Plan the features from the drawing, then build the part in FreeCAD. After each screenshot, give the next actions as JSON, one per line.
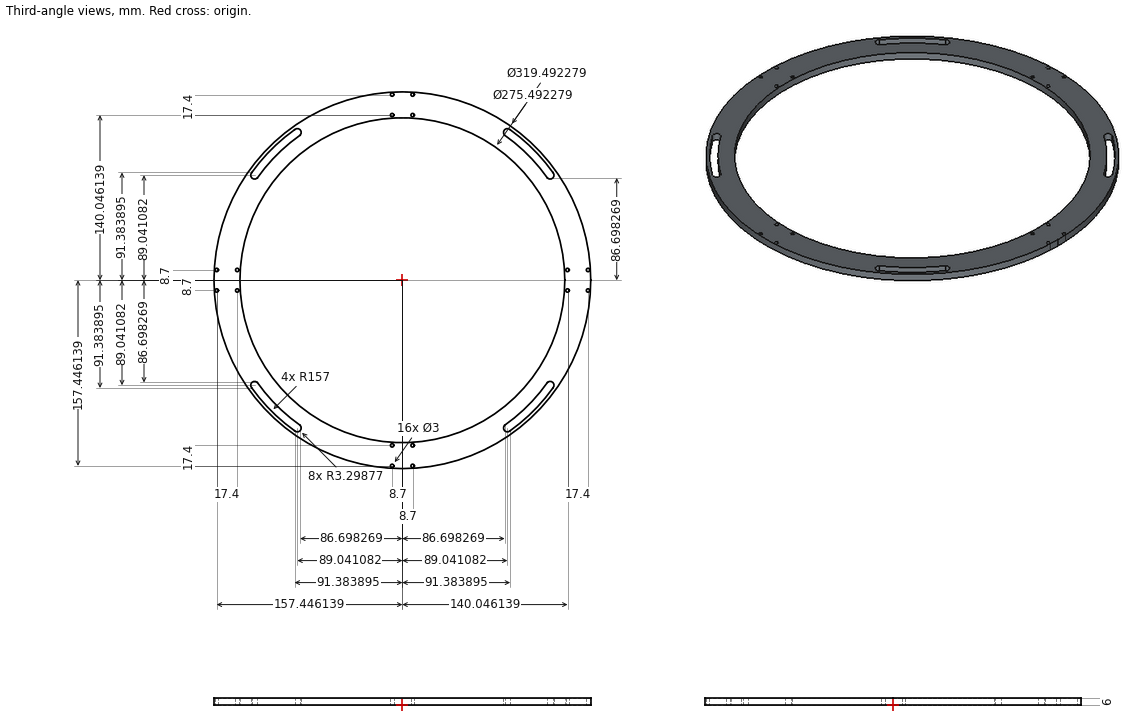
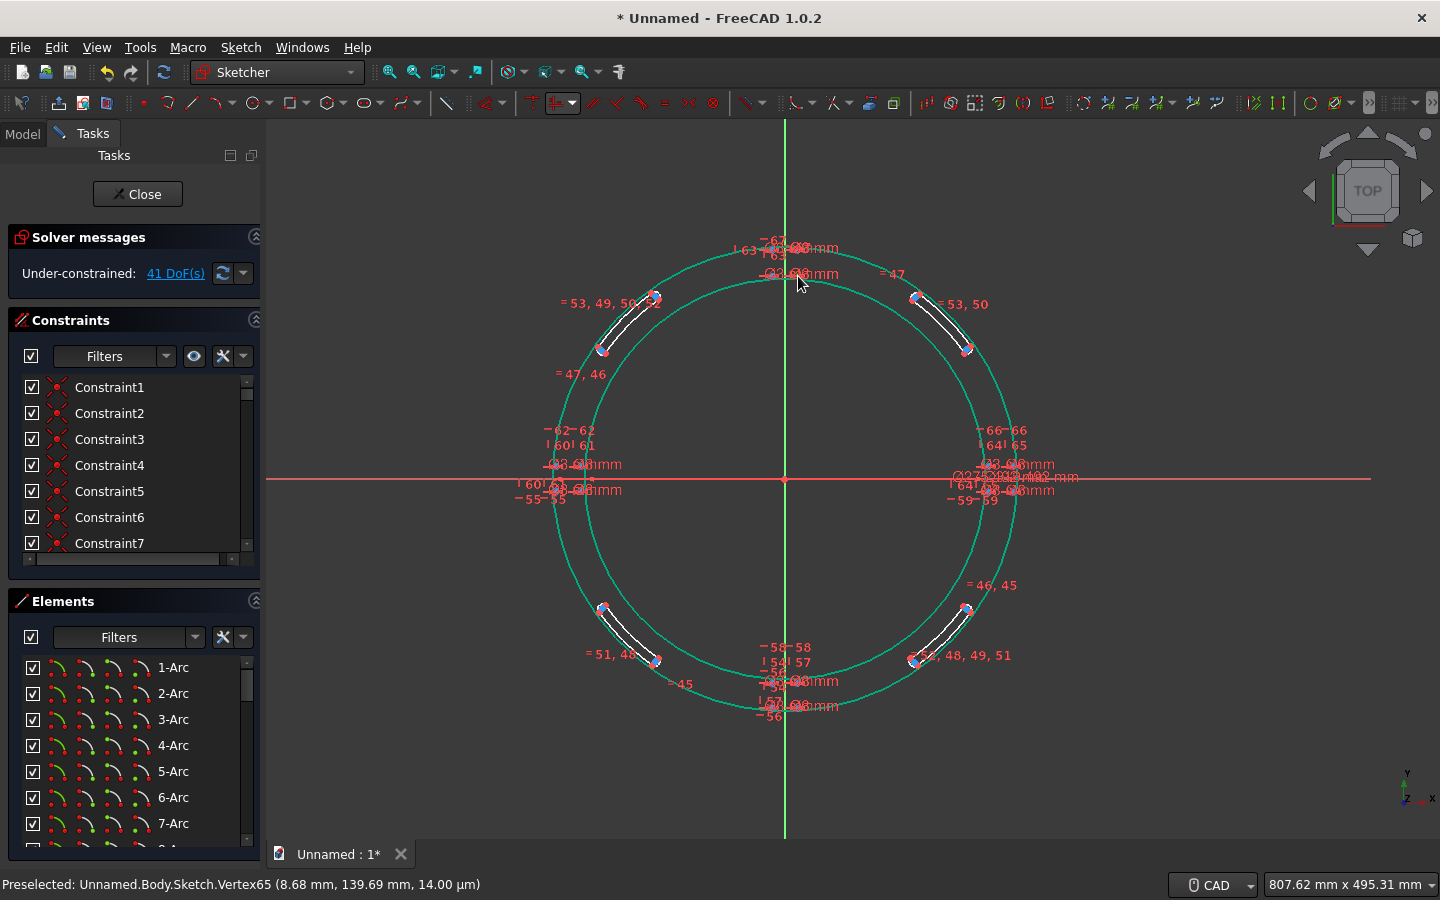
{"action": "scroll", "coordinate": [798, 250], "scroll_direction": "up", "scroll_amount": 4}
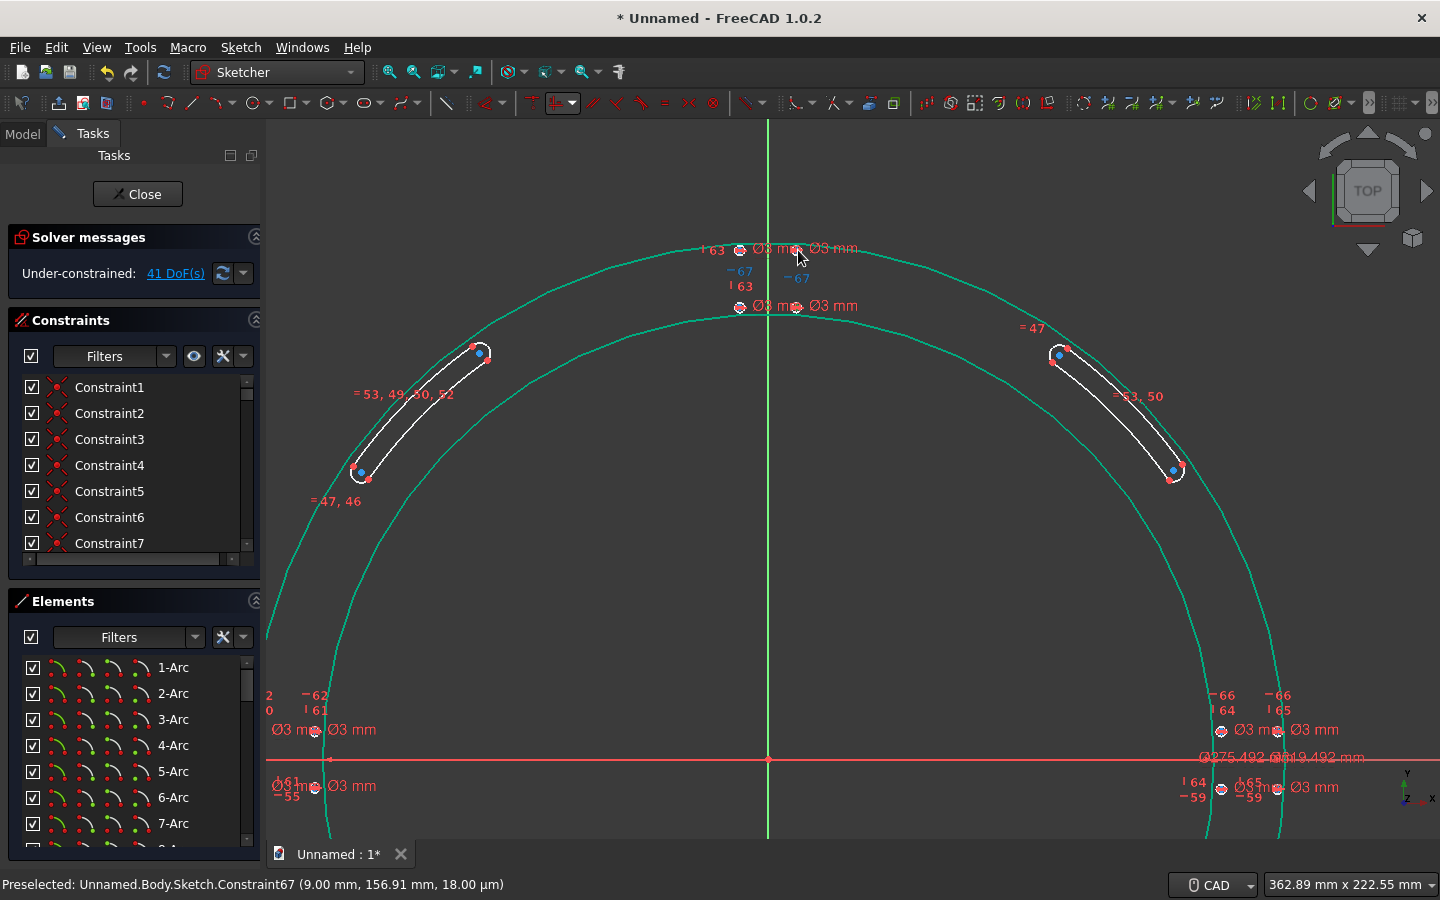
{"action": "left_click", "coordinate": [796, 250]}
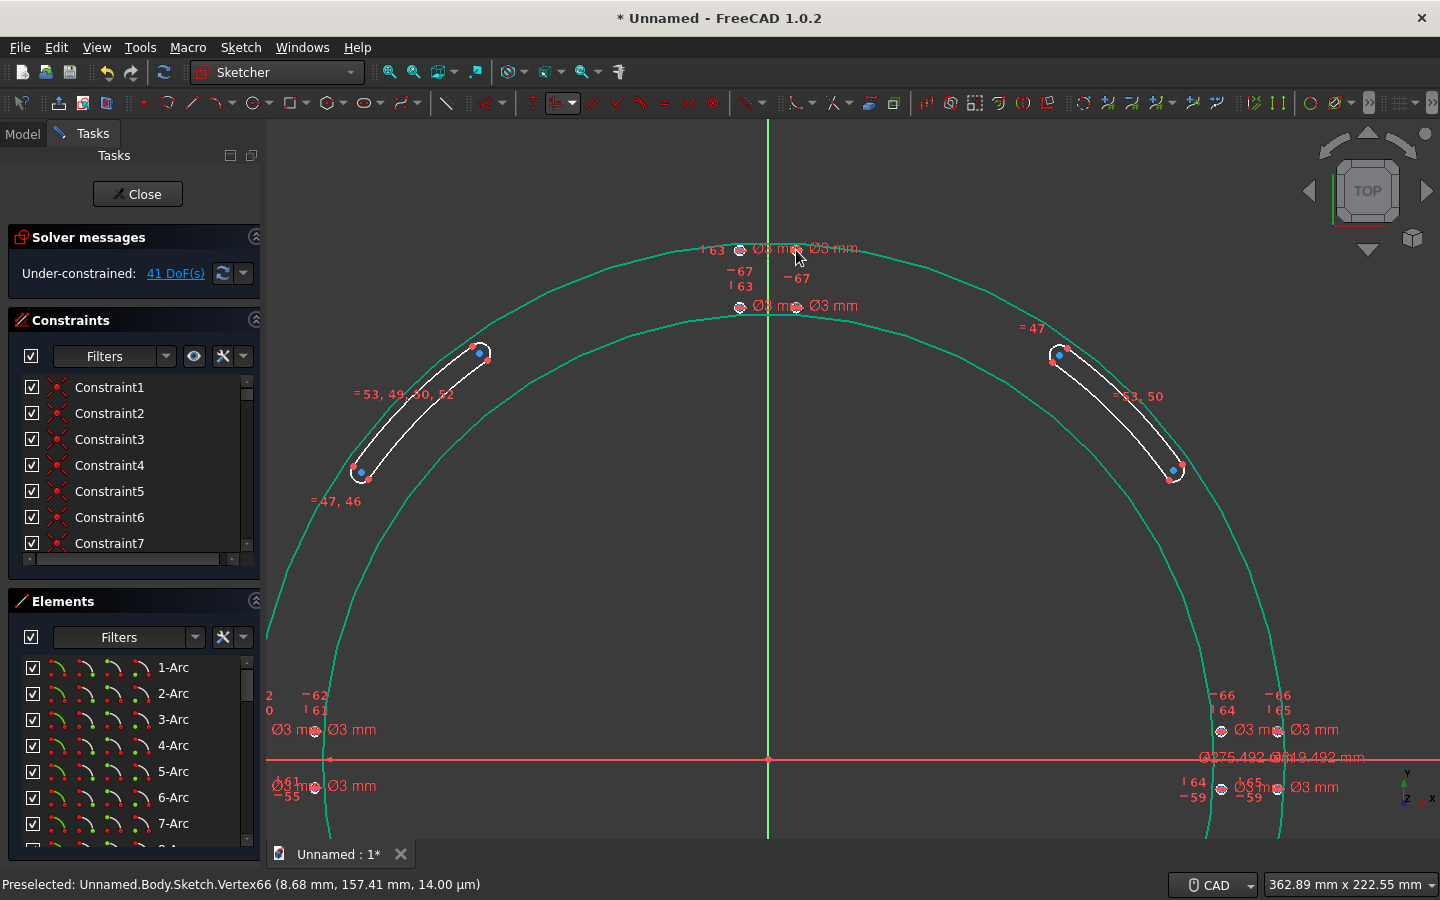
{"action": "key", "text": "v"}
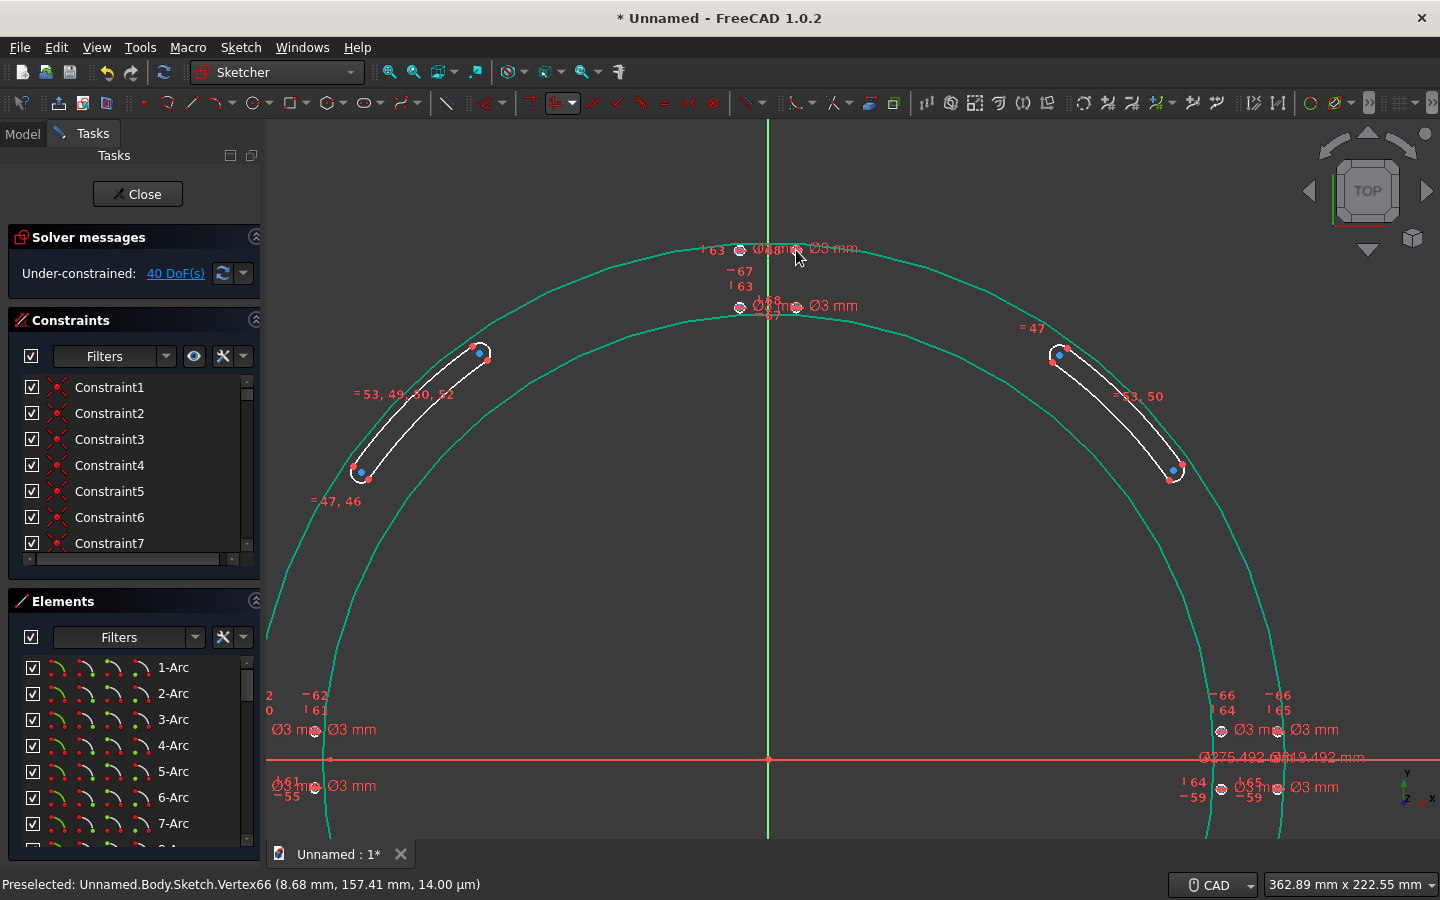
{"action": "left_click", "coordinate": [740, 251]}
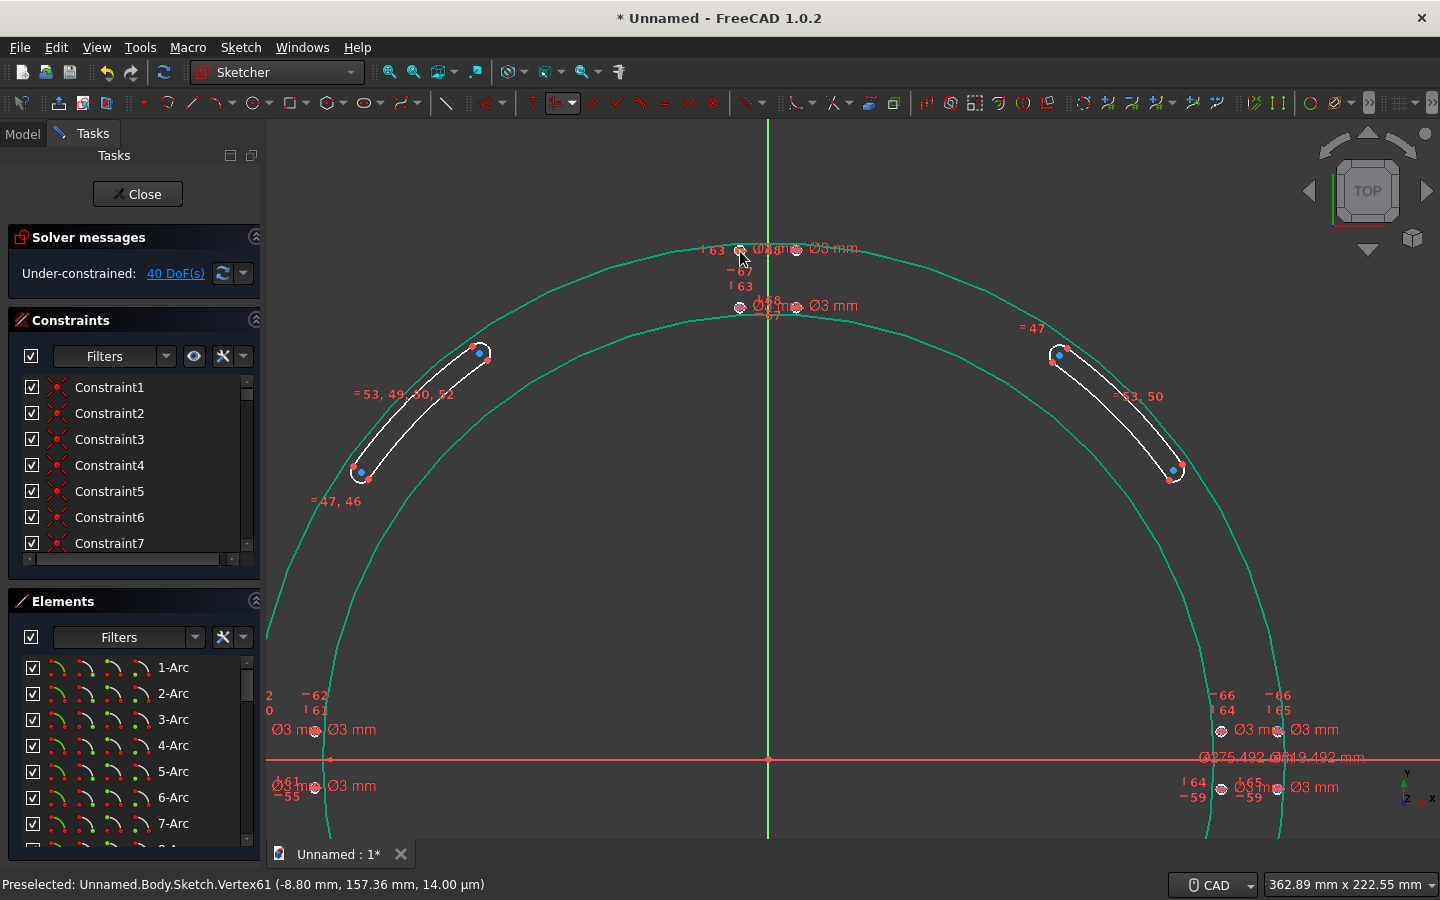
{"action": "left_click", "coordinate": [796, 250]}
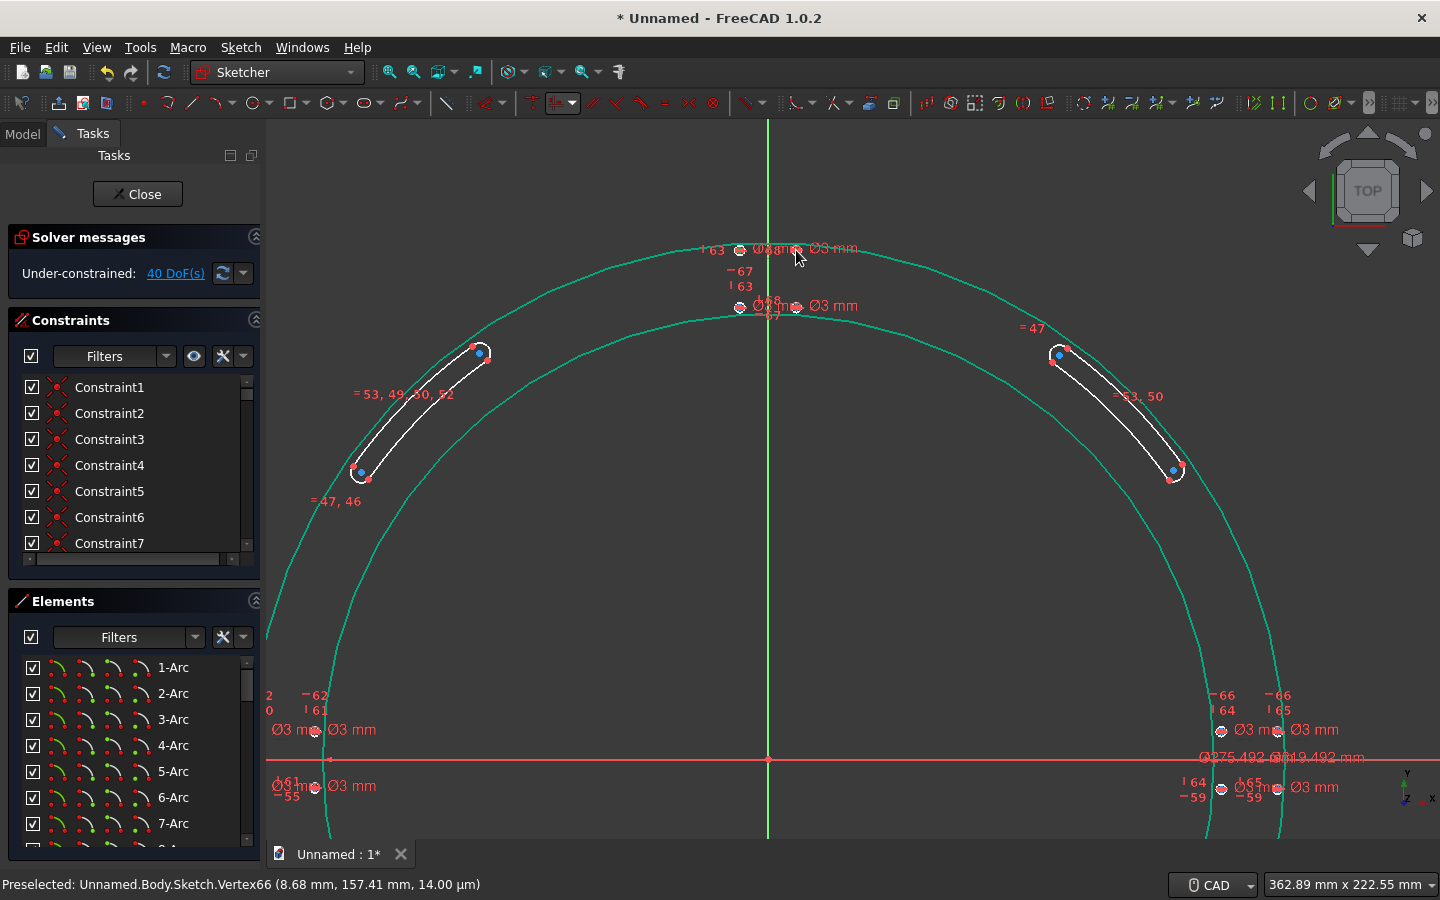
{"action": "key", "text": "h"}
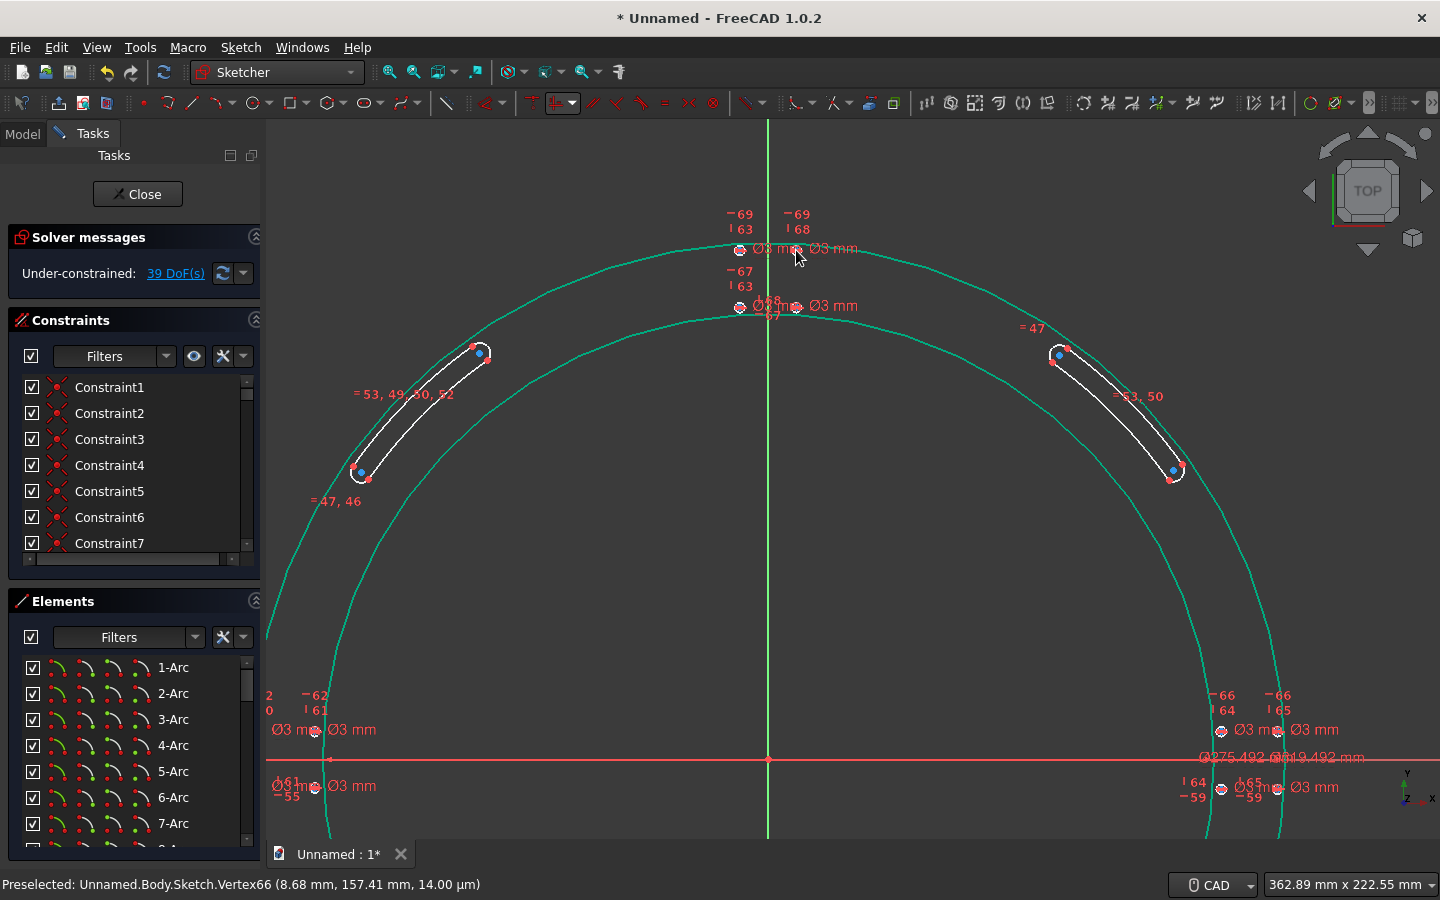
{"action": "left_click", "coordinate": [486, 104]}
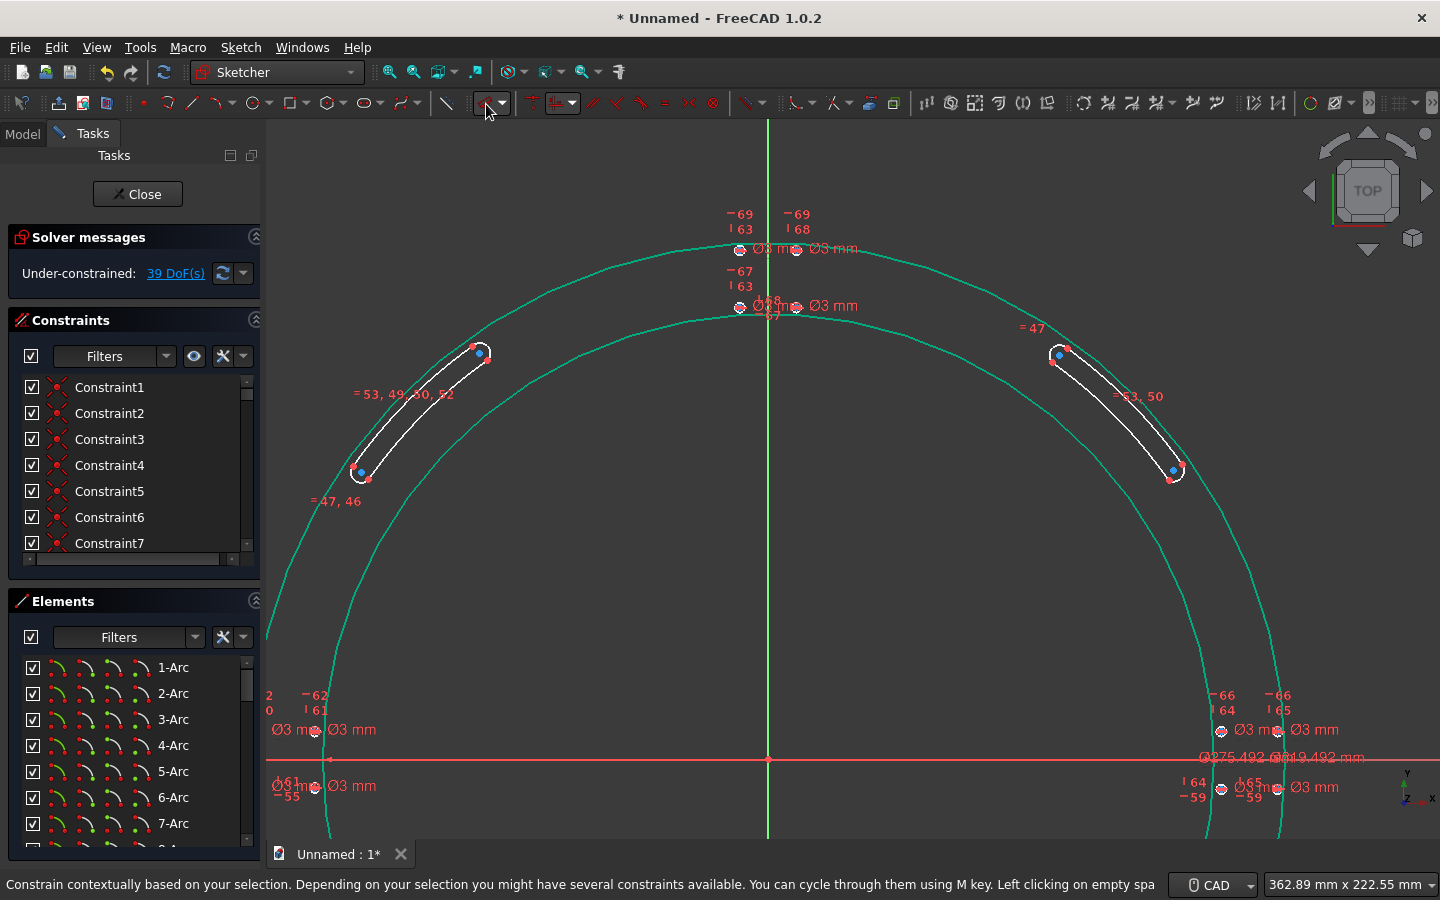
{"action": "scroll", "coordinate": [798, 250], "scroll_direction": "down", "scroll_amount": 4}